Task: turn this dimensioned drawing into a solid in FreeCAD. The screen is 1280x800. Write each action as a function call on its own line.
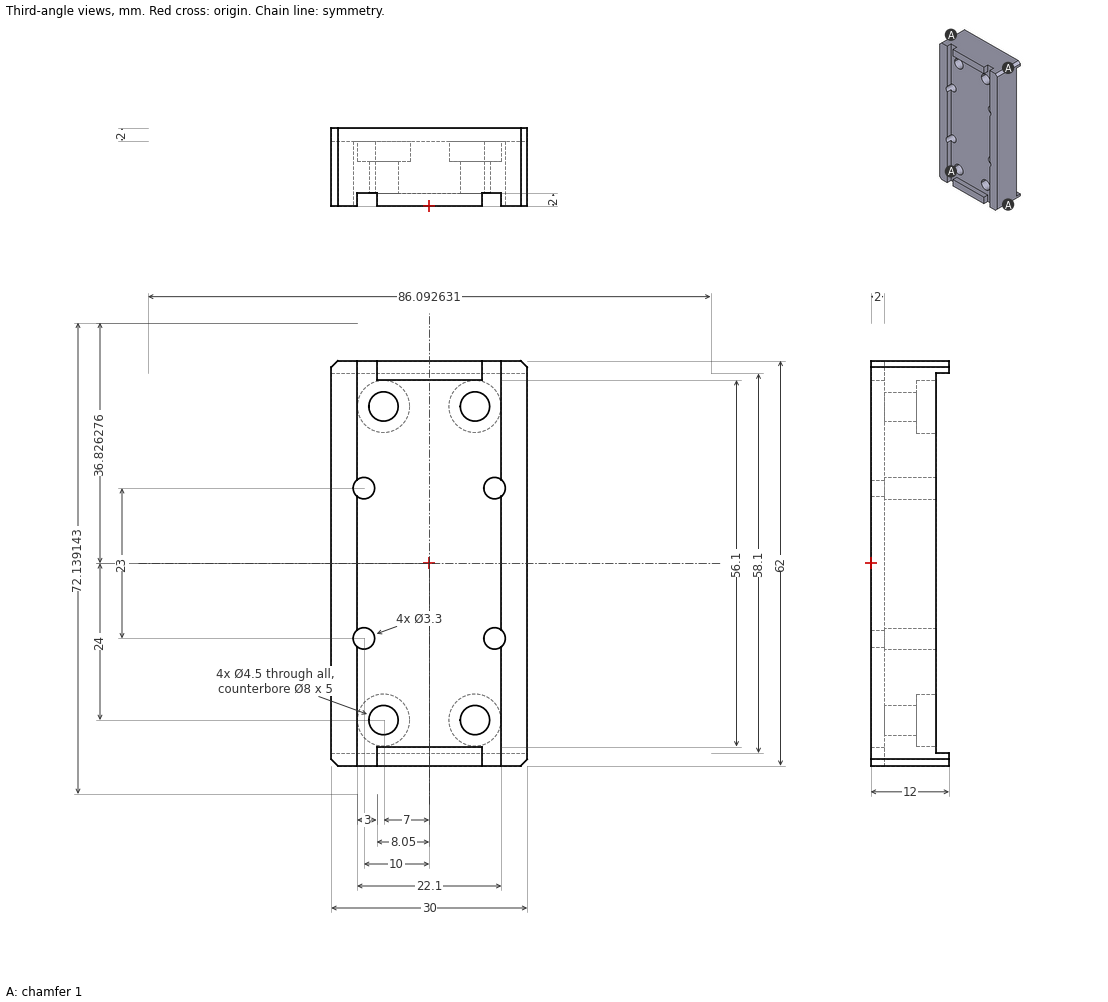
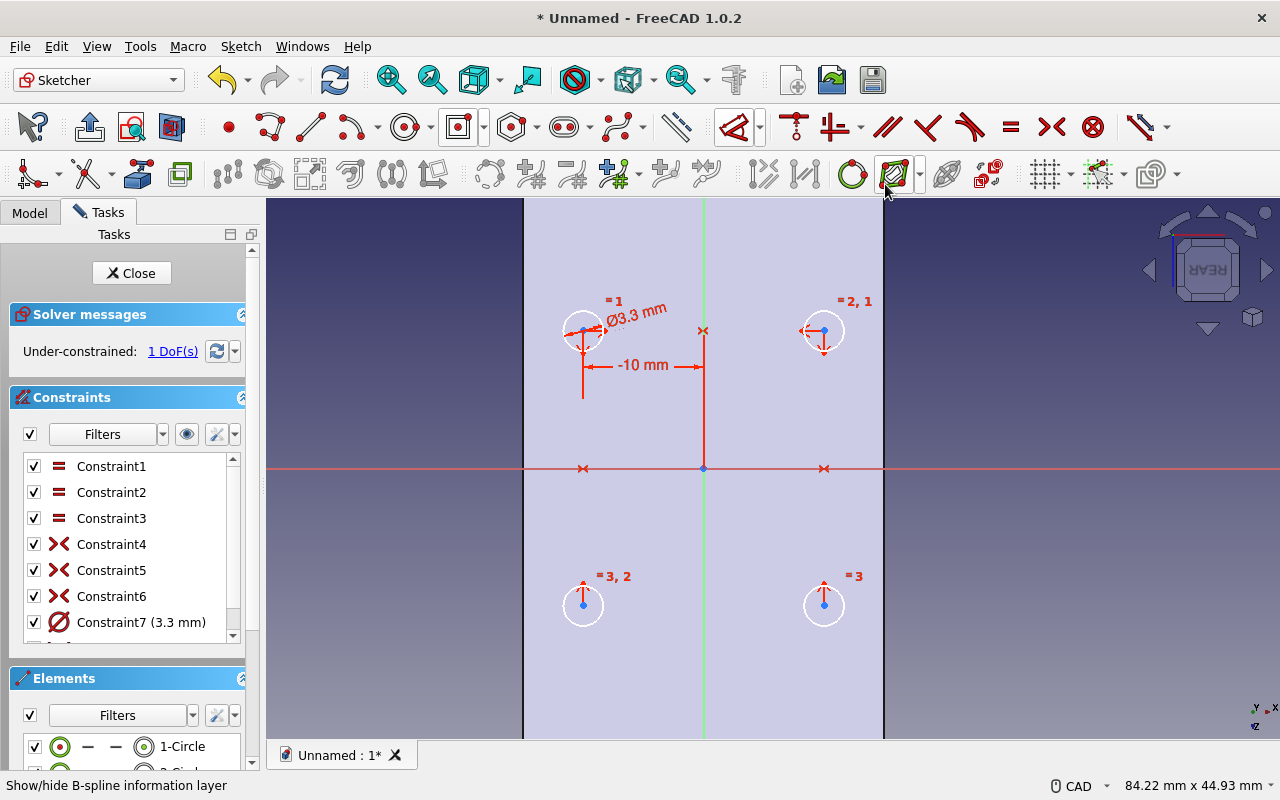
click(583, 331)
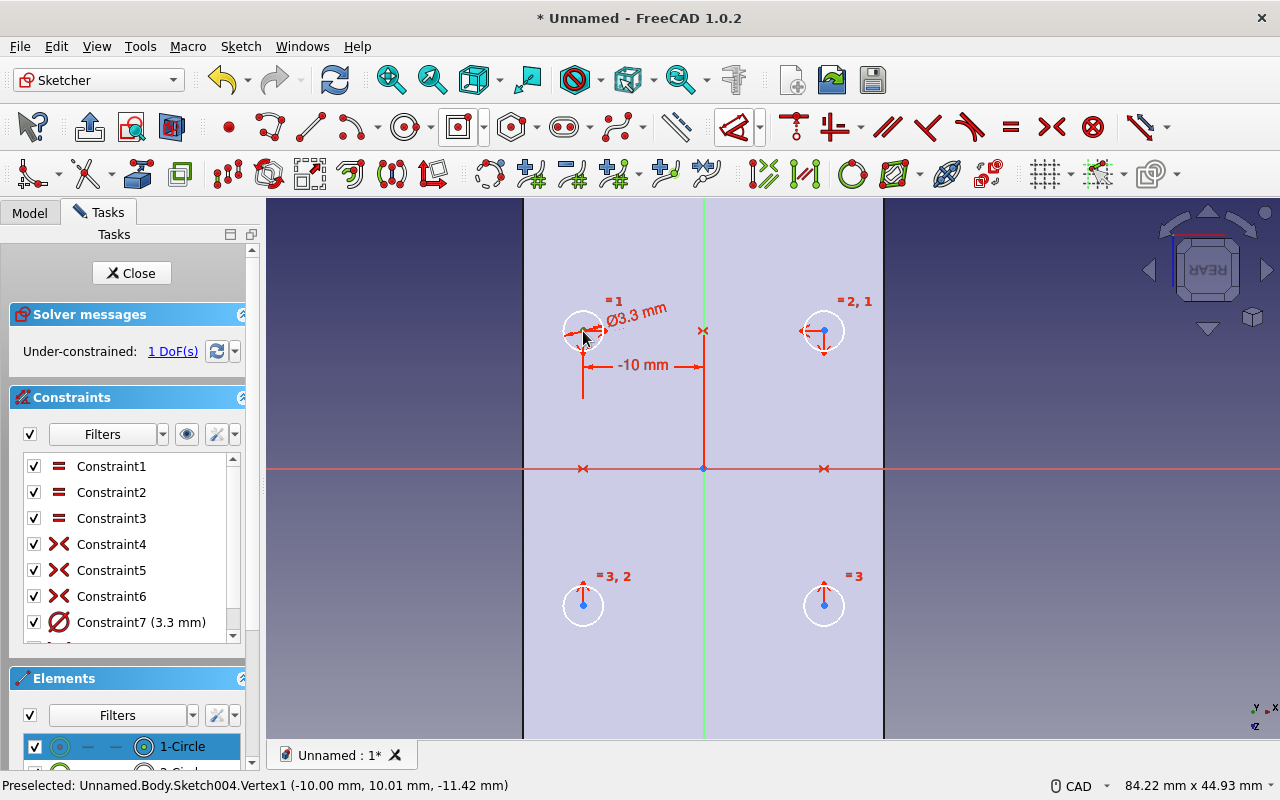
click(583, 606)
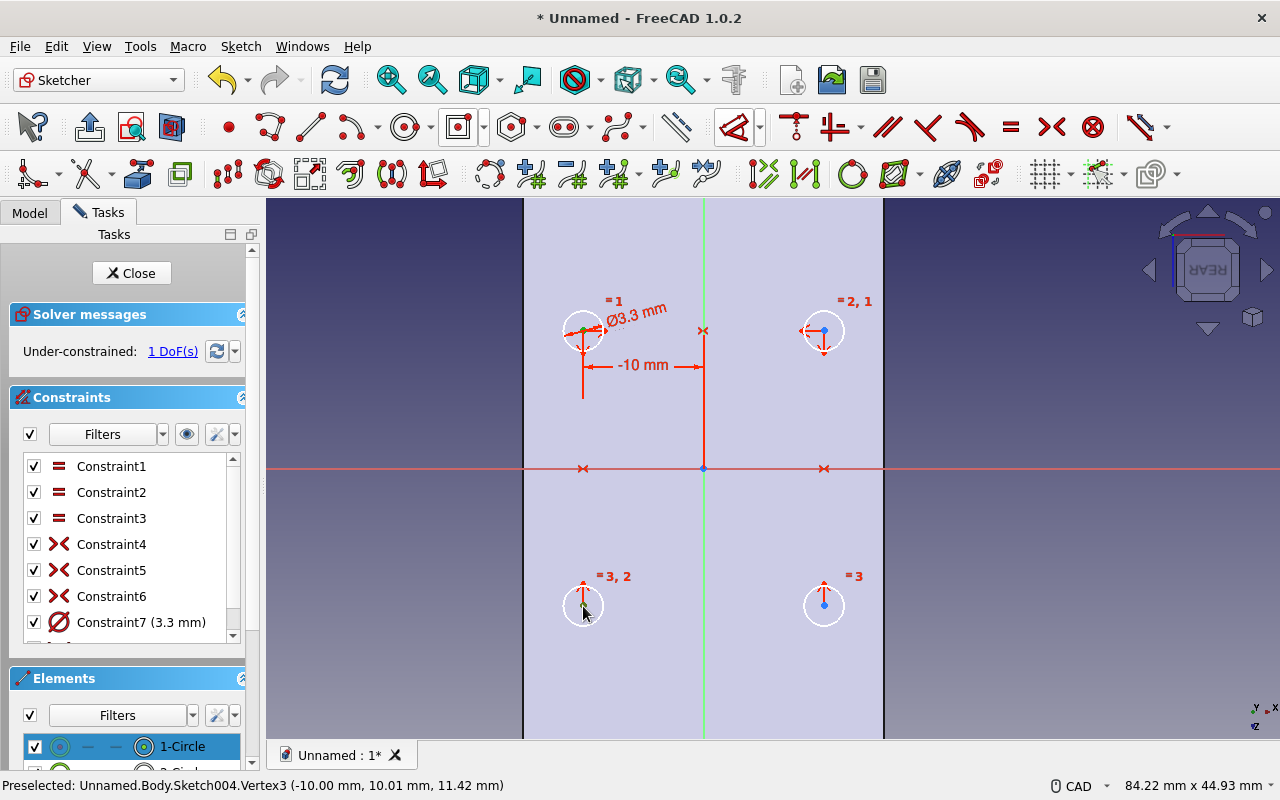
click(760, 128)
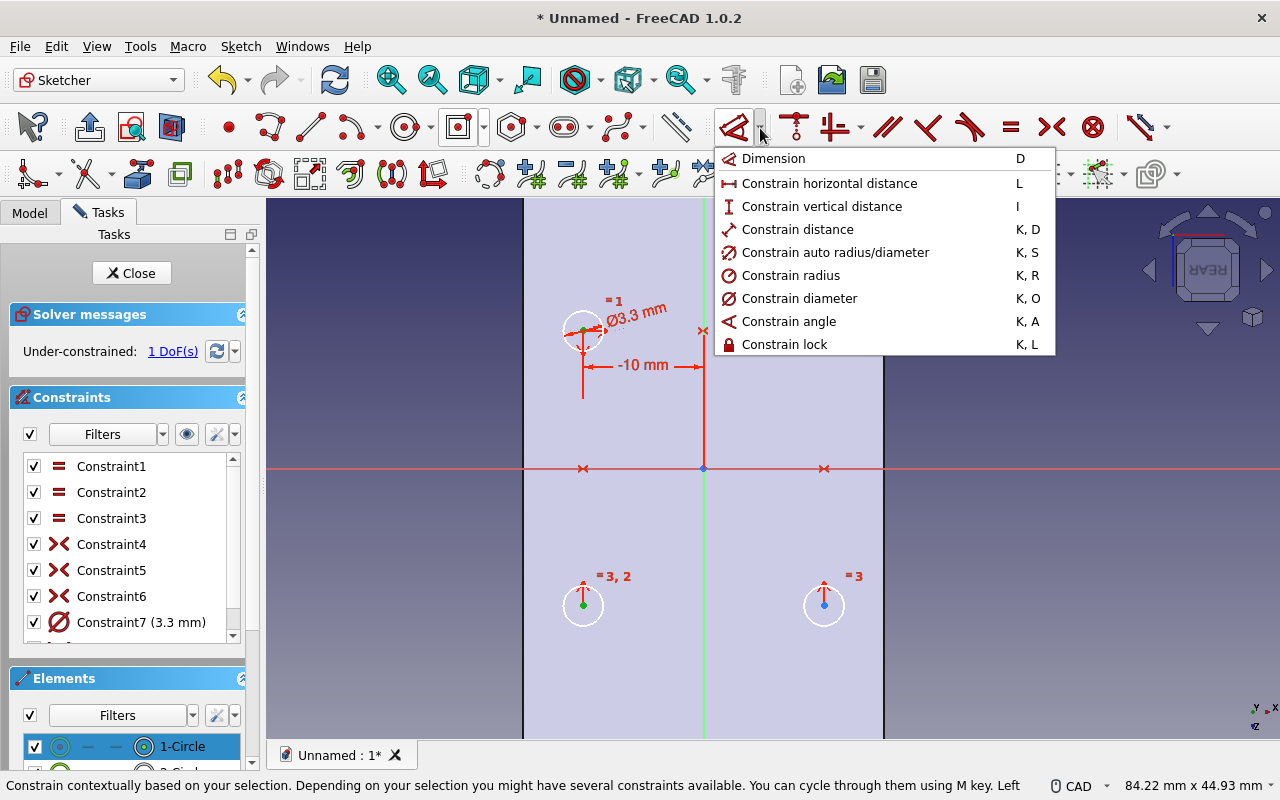
click(885, 206)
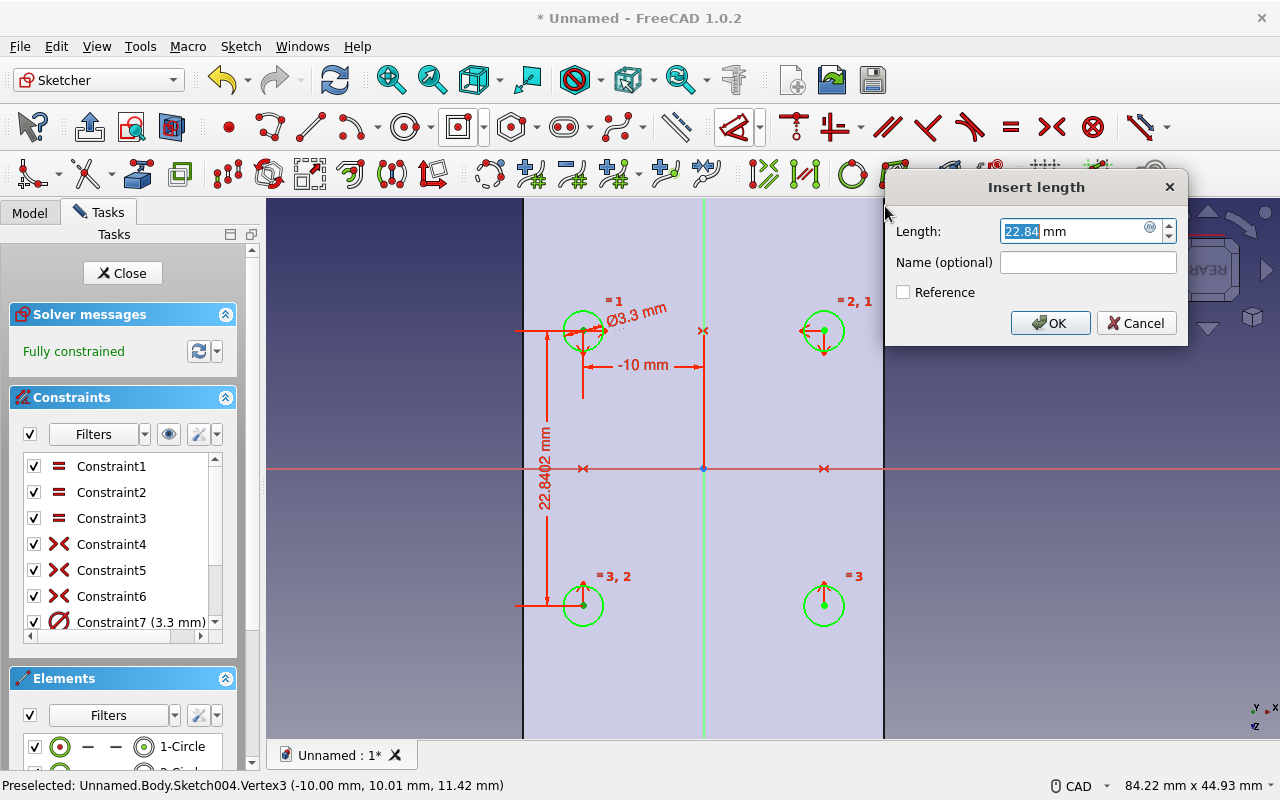
text(23)
key(Return)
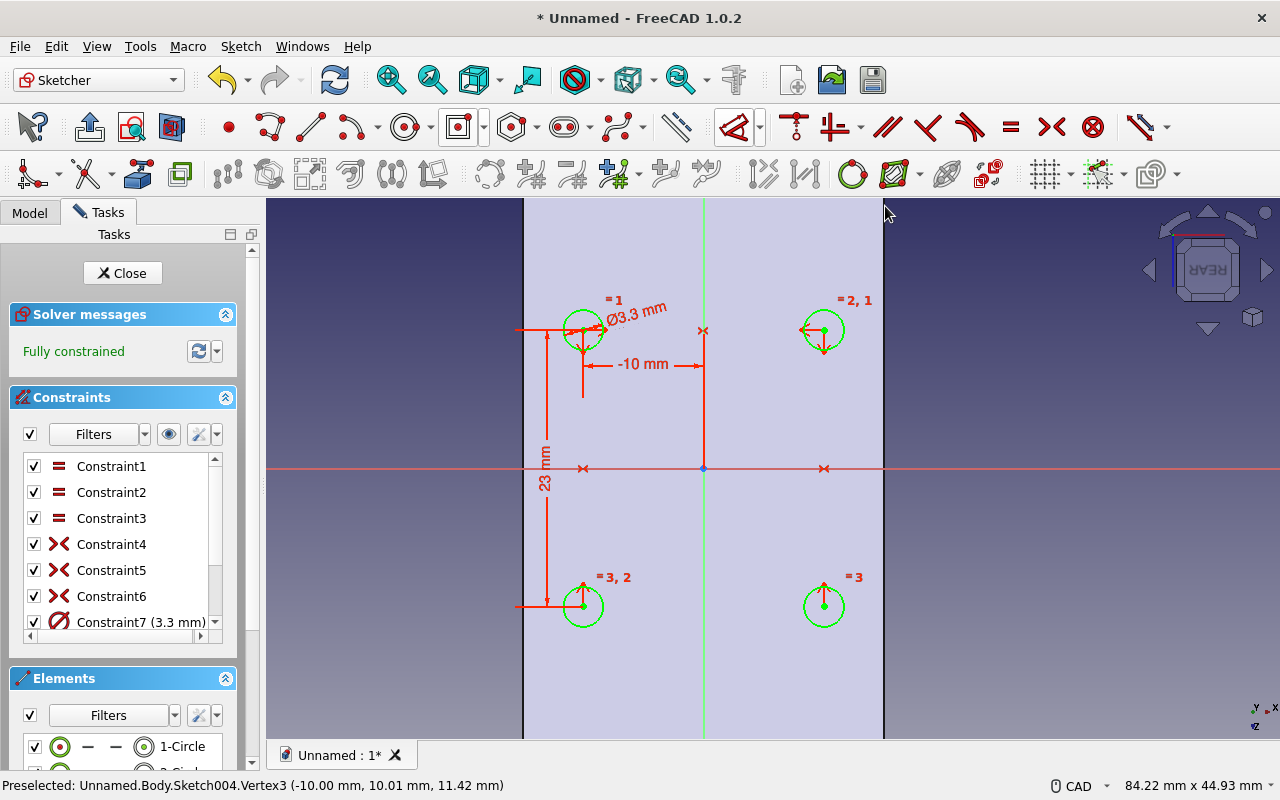
click(123, 273)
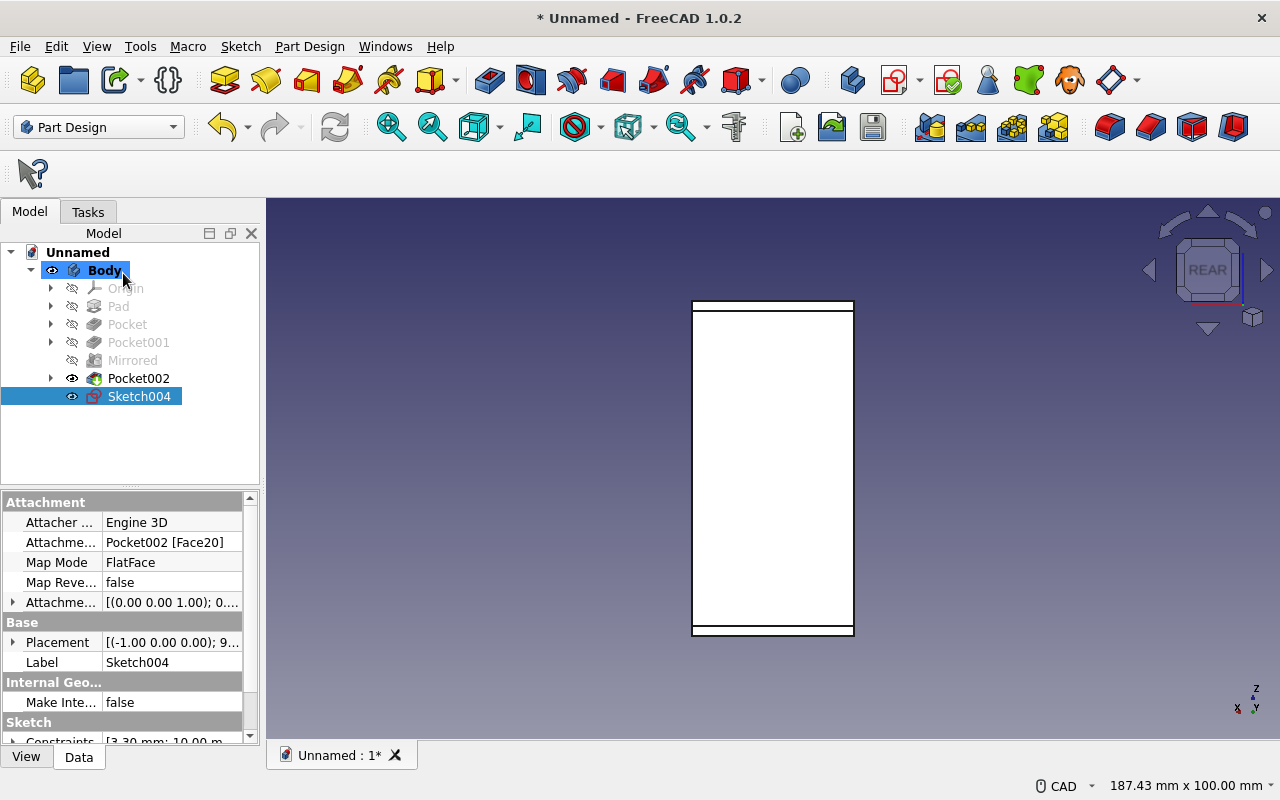
click(490, 80)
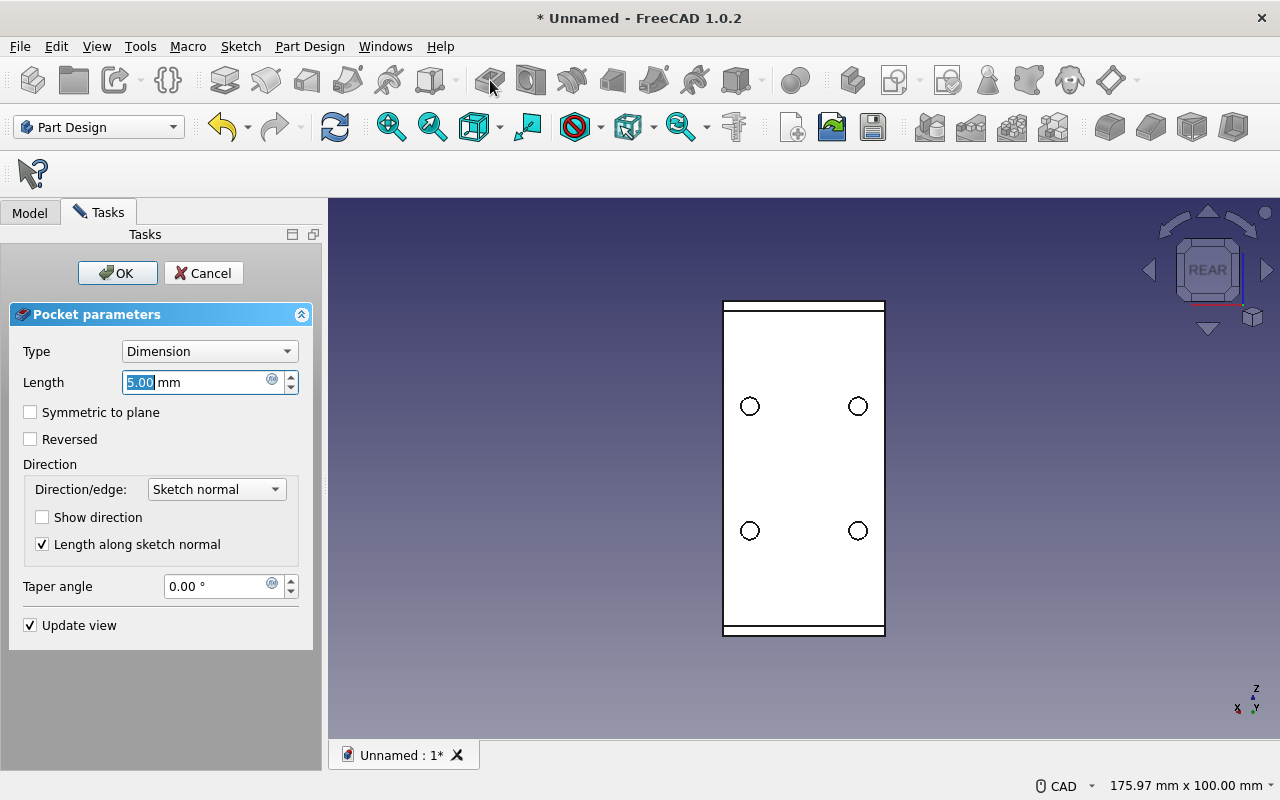
click(210, 352)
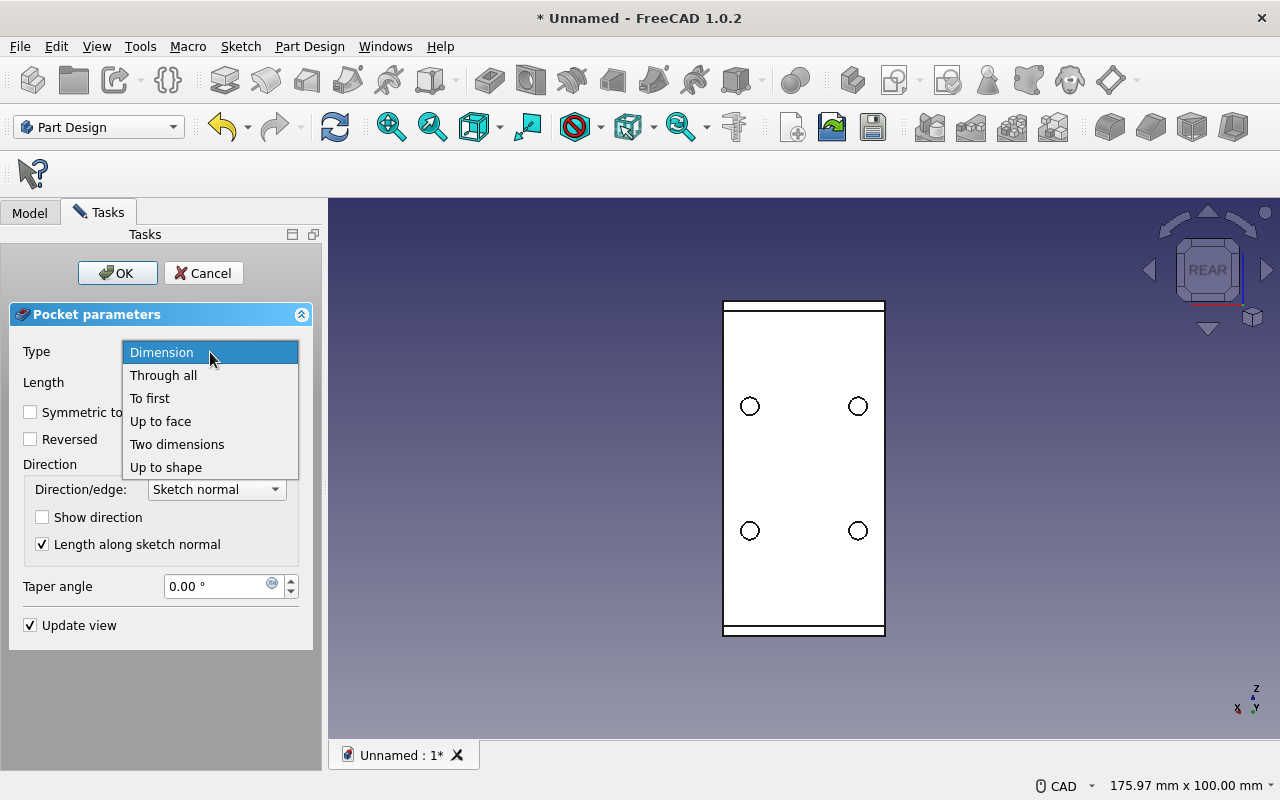
click(208, 376)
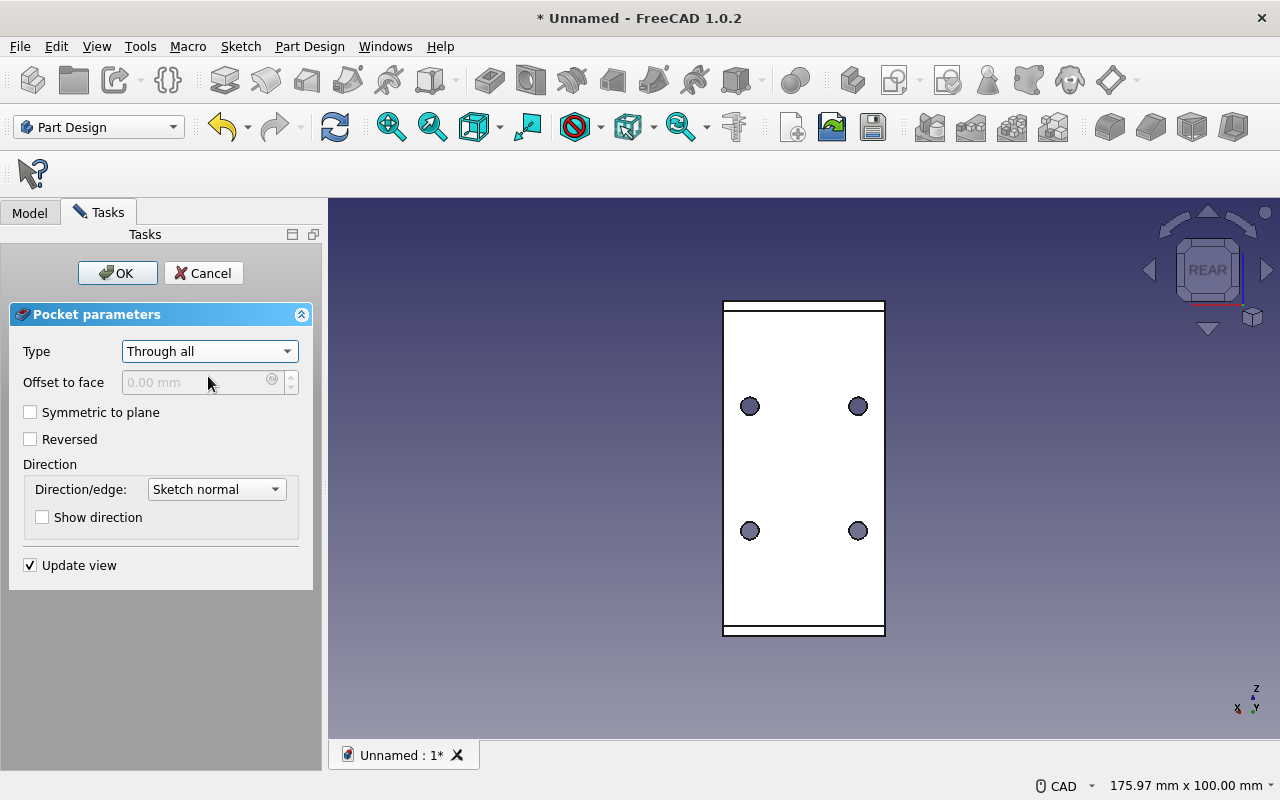
click(118, 273)